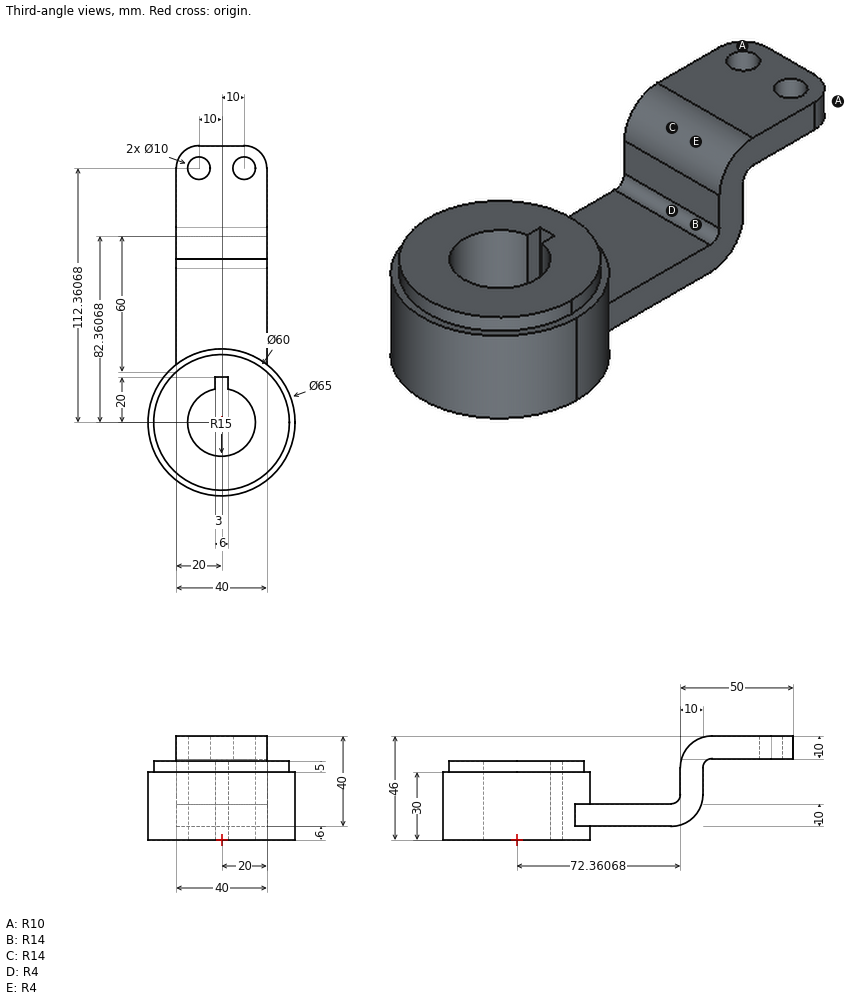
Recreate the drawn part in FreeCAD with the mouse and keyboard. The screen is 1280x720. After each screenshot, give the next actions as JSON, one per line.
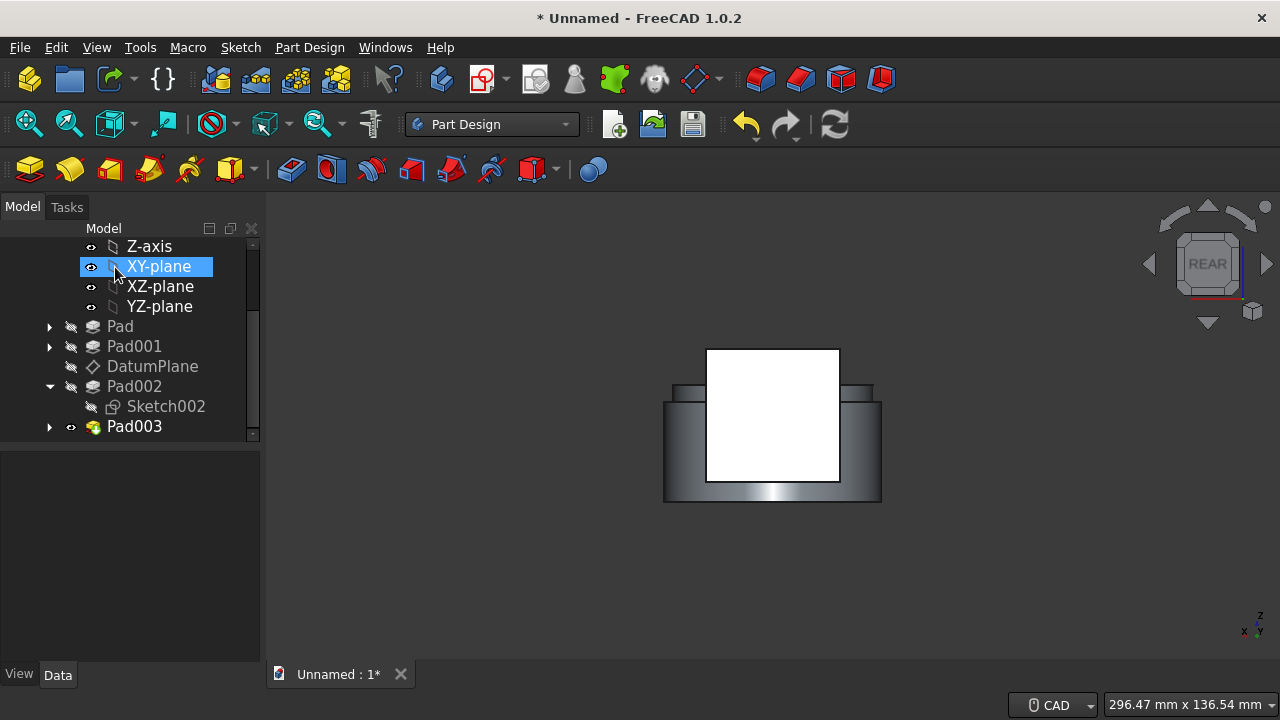
{"action": "key", "text": "0"}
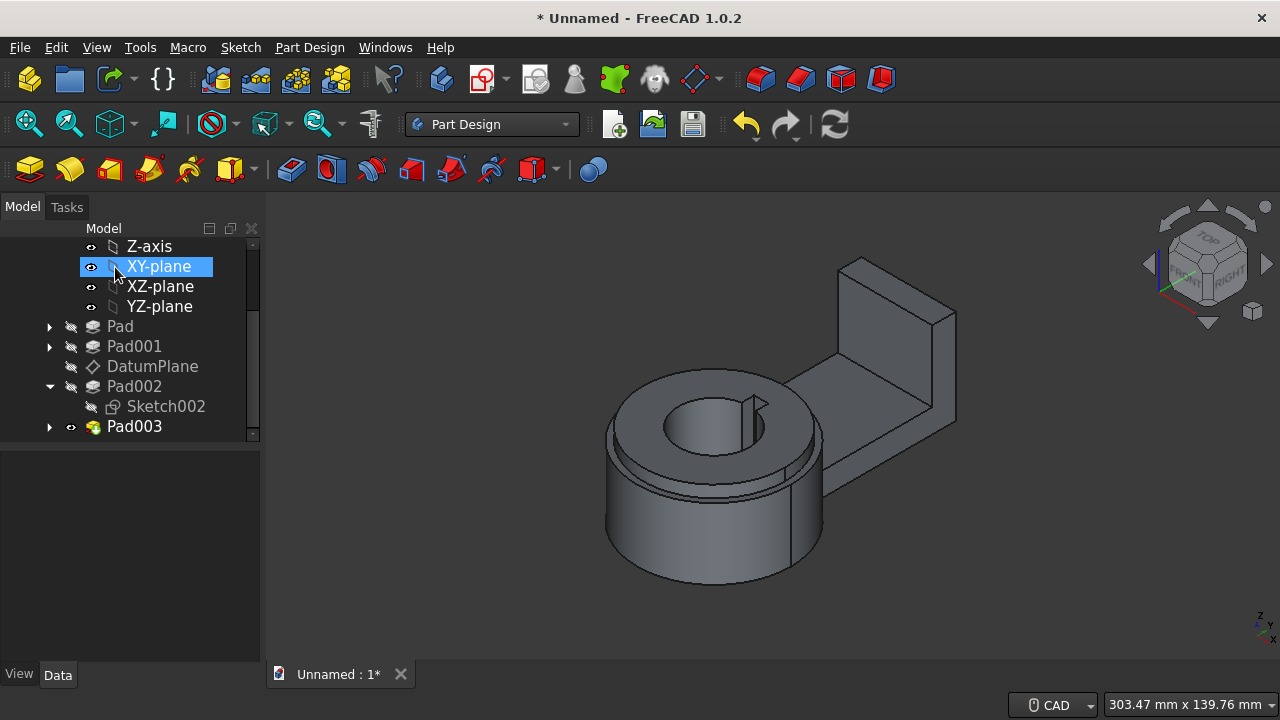
{"action": "left_click", "coordinate": [946, 340]}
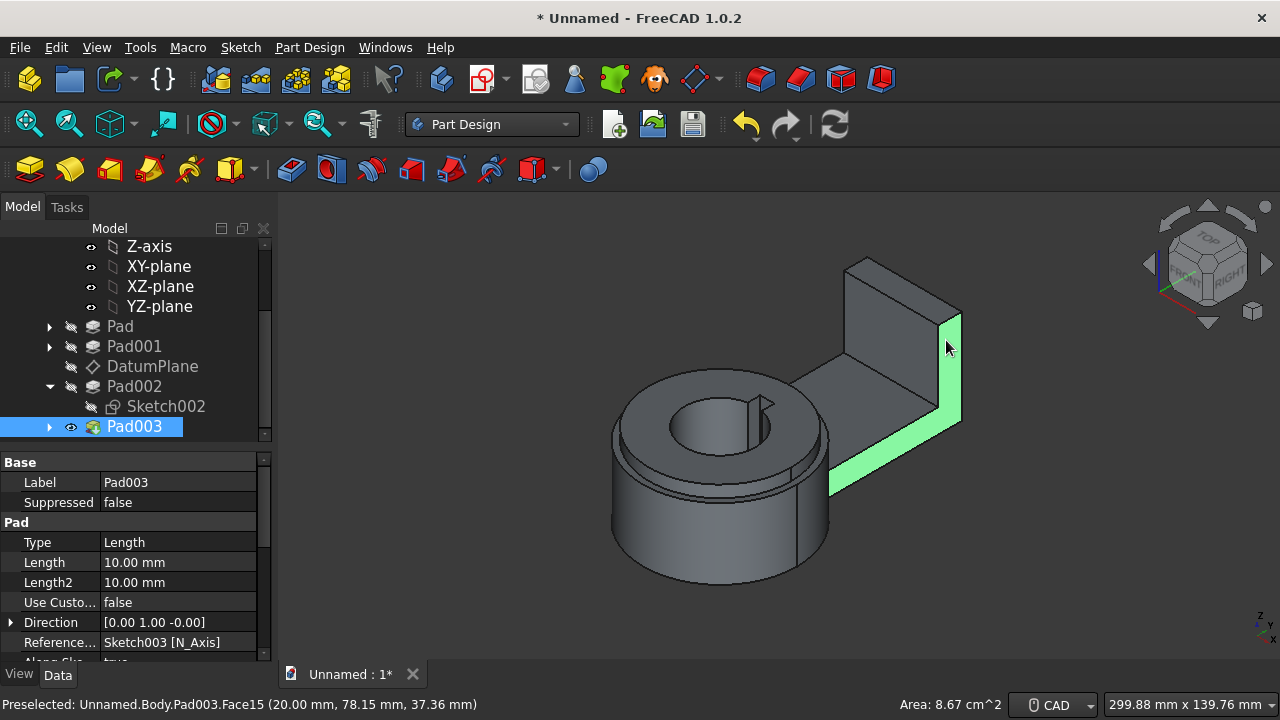
{"action": "left_click", "coordinate": [482, 80]}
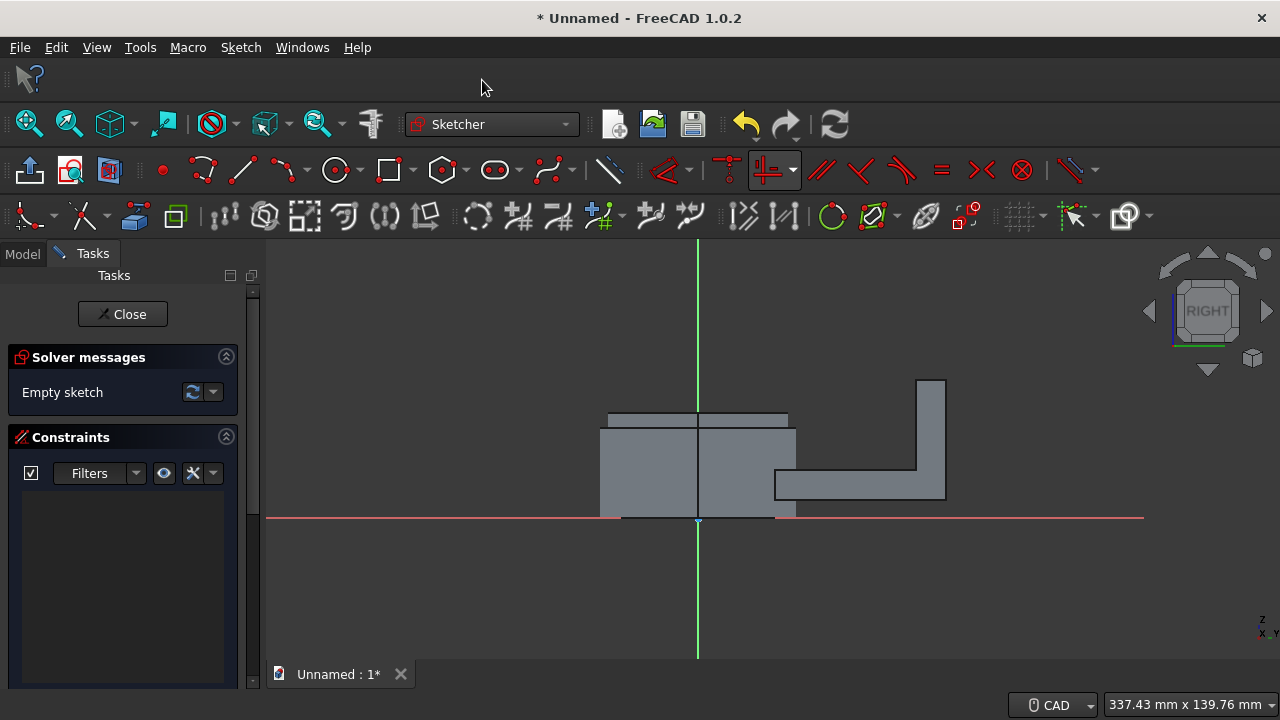
{"action": "scroll", "coordinate": [1115, 449], "scroll_direction": "up", "scroll_amount": 2}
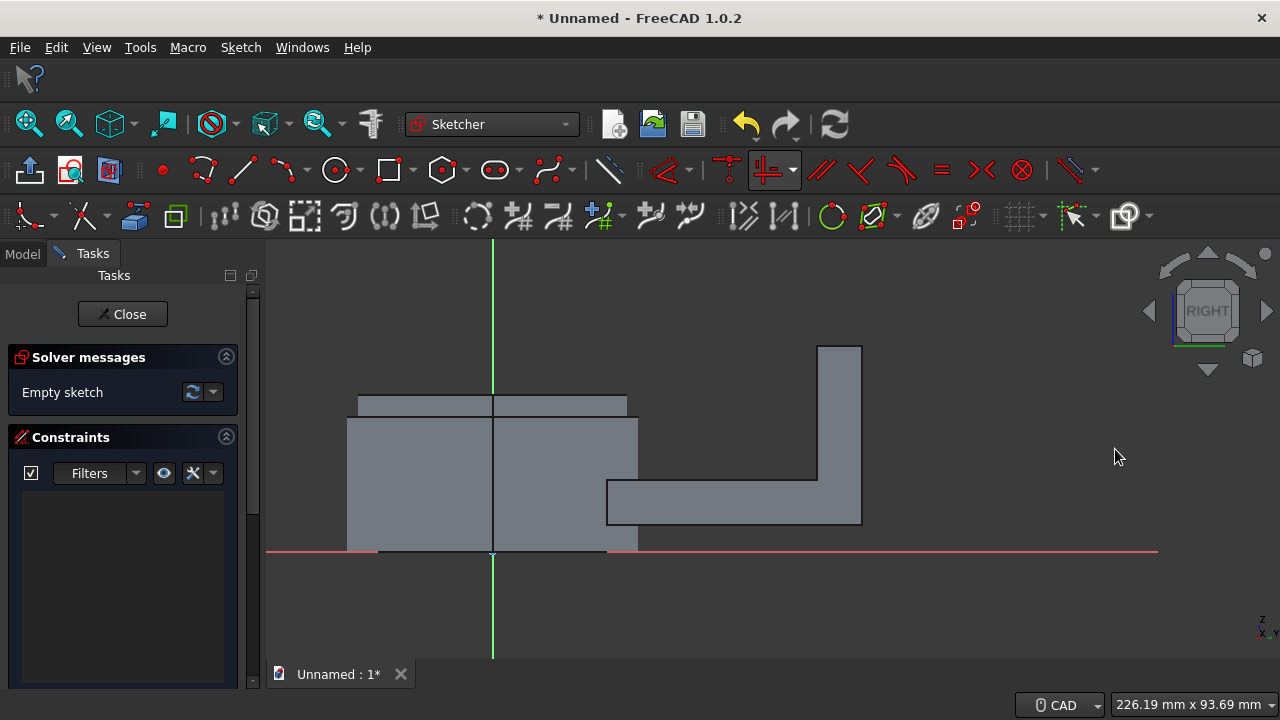
{"action": "key", "text": "g r"}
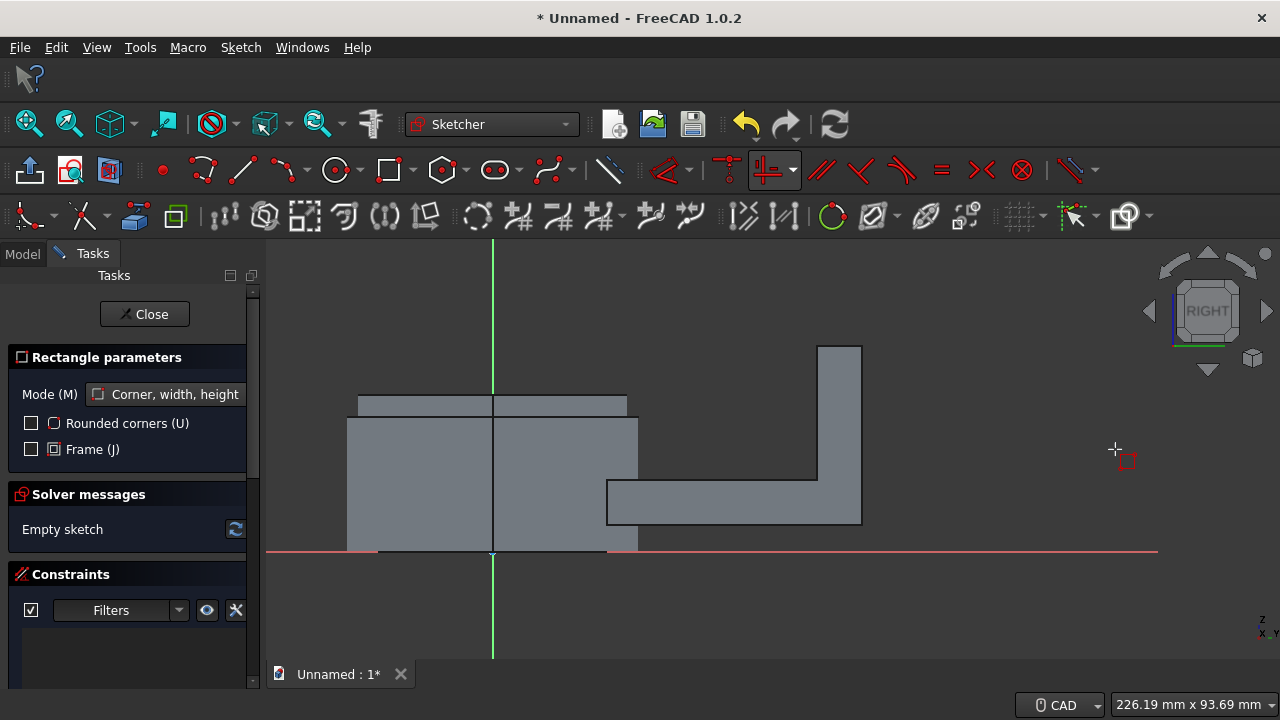
{"action": "left_click", "coordinate": [817, 346]}
{"action": "left_click", "coordinate": [1041, 390]}
{"action": "key", "text": "Escape"}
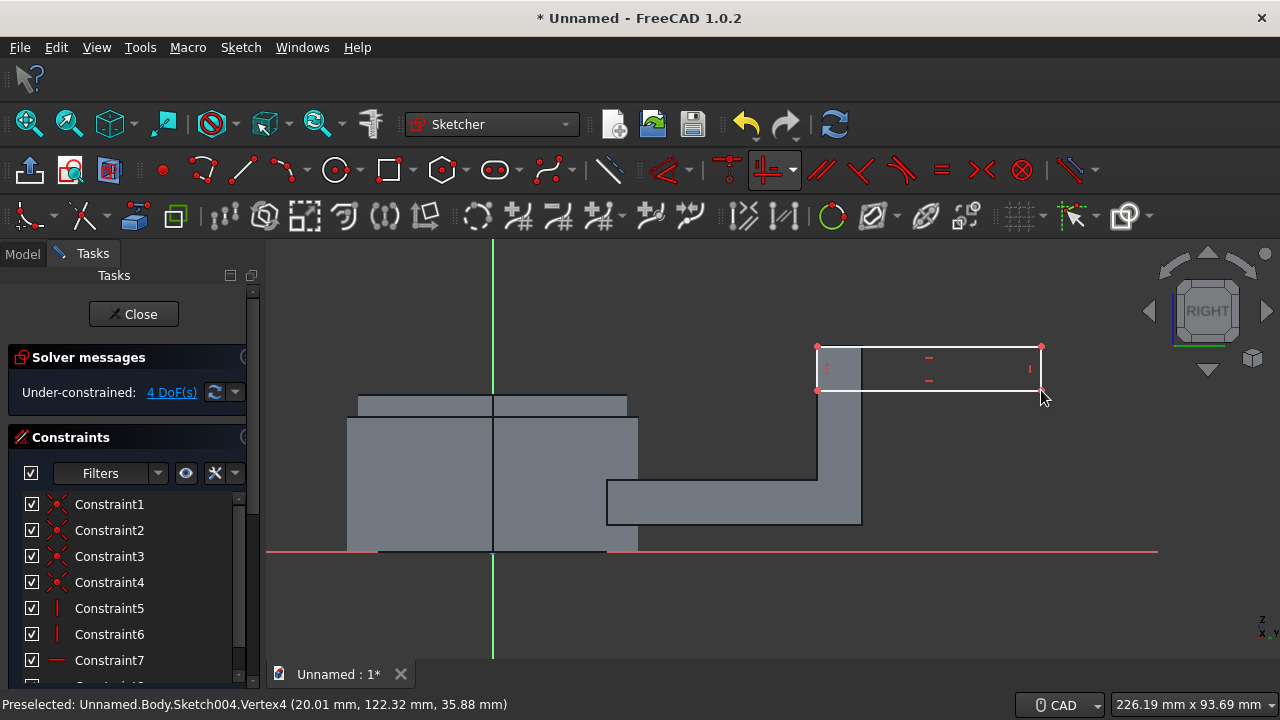
{"action": "key", "text": "d"}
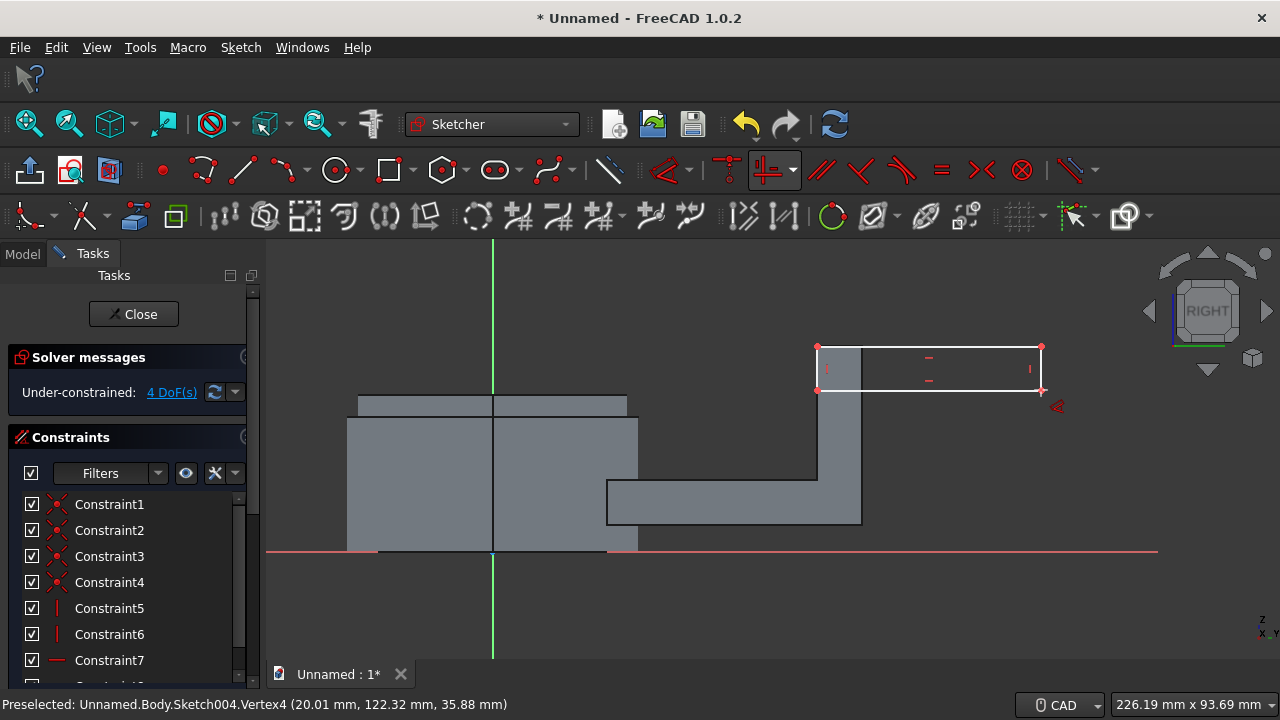
{"action": "left_click", "coordinate": [817, 360]}
{"action": "left_click", "coordinate": [851, 369]}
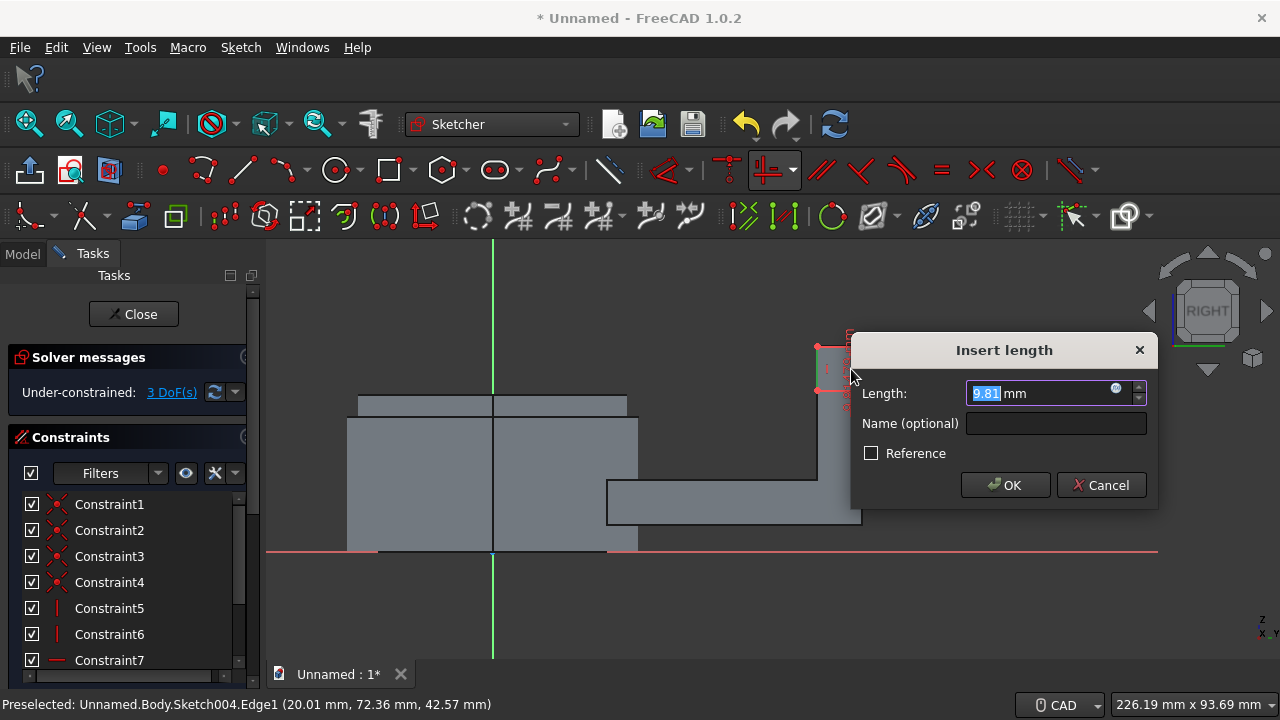
{"action": "type", "text": "10"}
{"action": "key", "text": "Return"}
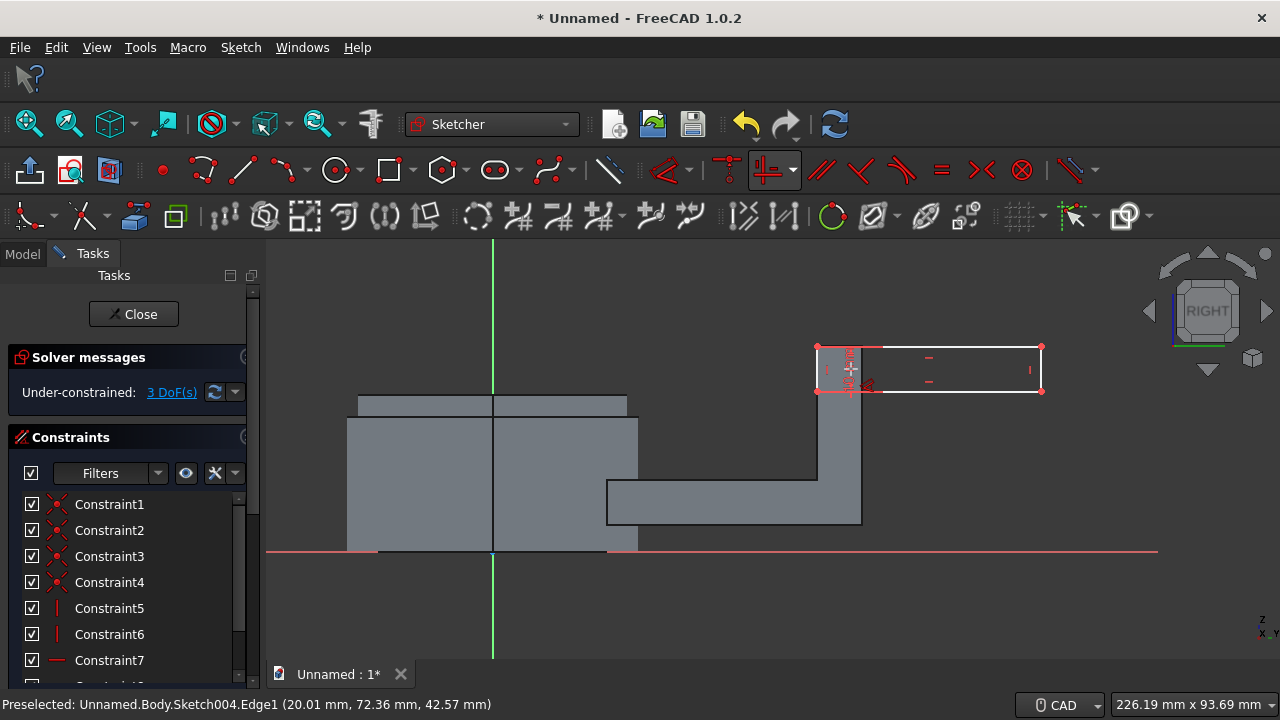
{"action": "left_click", "coordinate": [884, 392]}
{"action": "left_click", "coordinate": [929, 426]}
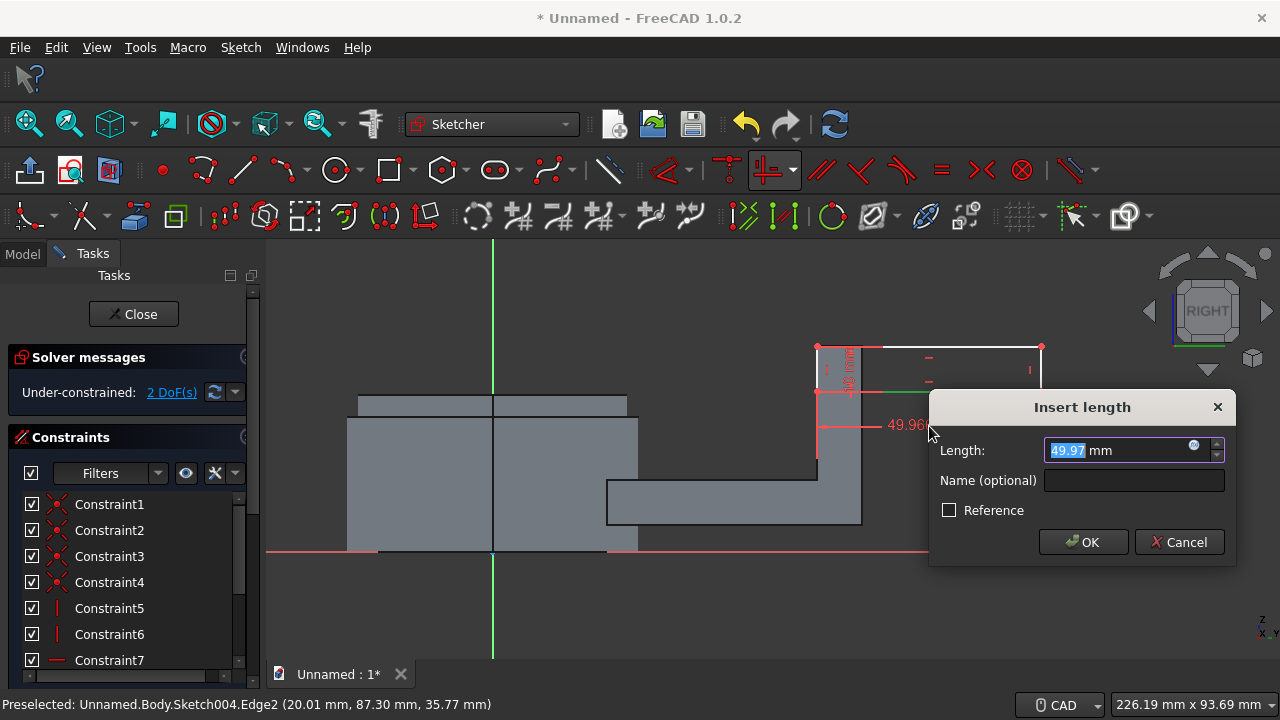
{"action": "type", "text": "50"}
{"action": "key", "text": "Return"}